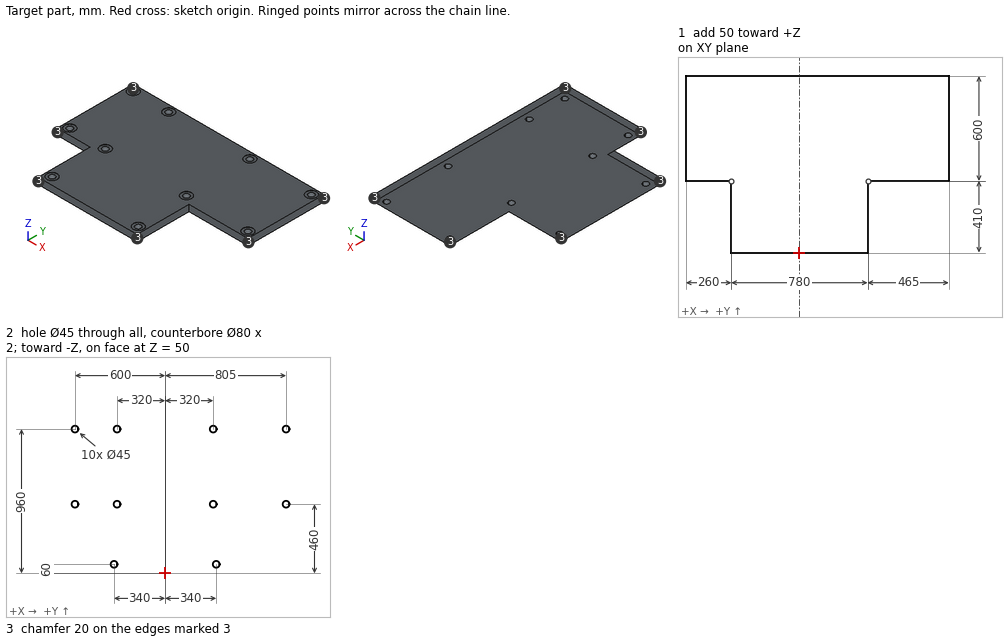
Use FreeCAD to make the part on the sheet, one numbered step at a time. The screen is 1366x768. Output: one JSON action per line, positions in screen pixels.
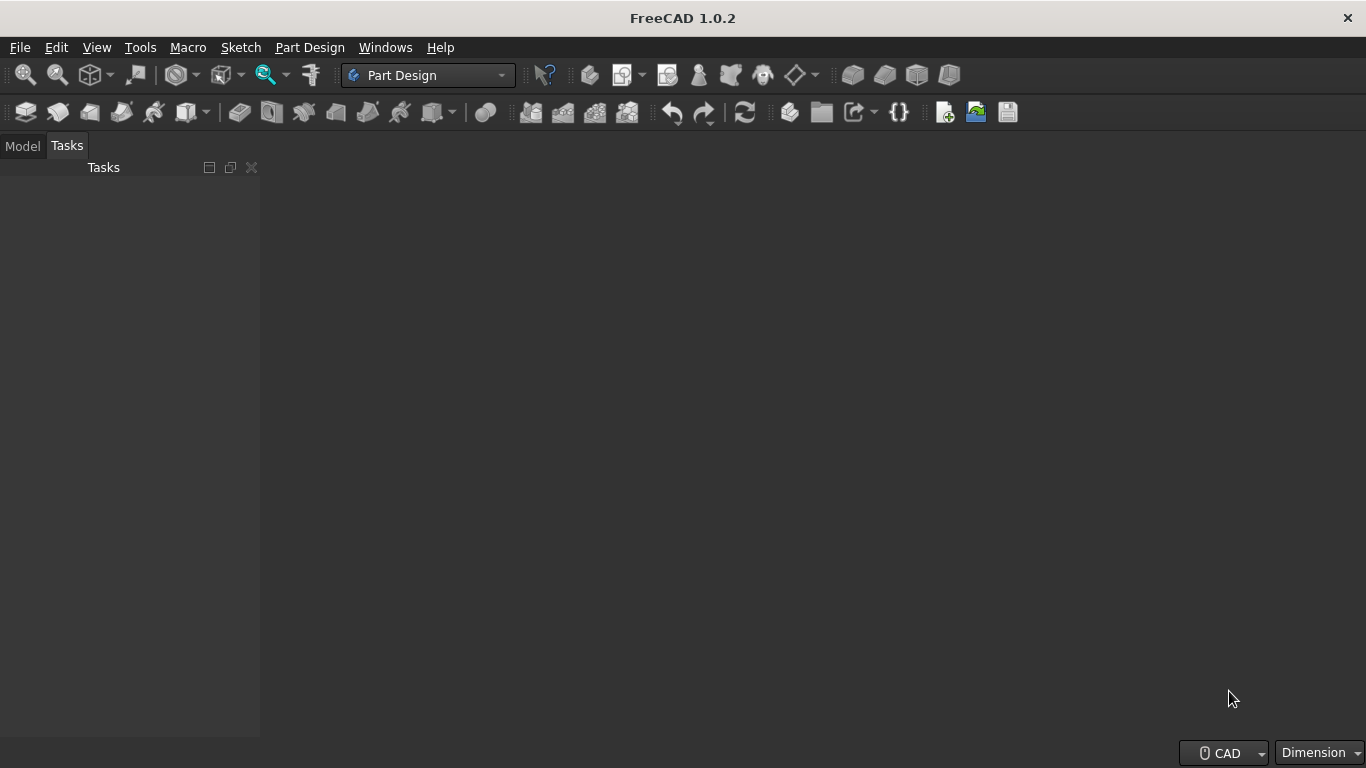
{"action": "left_click", "coordinate": [944, 112]}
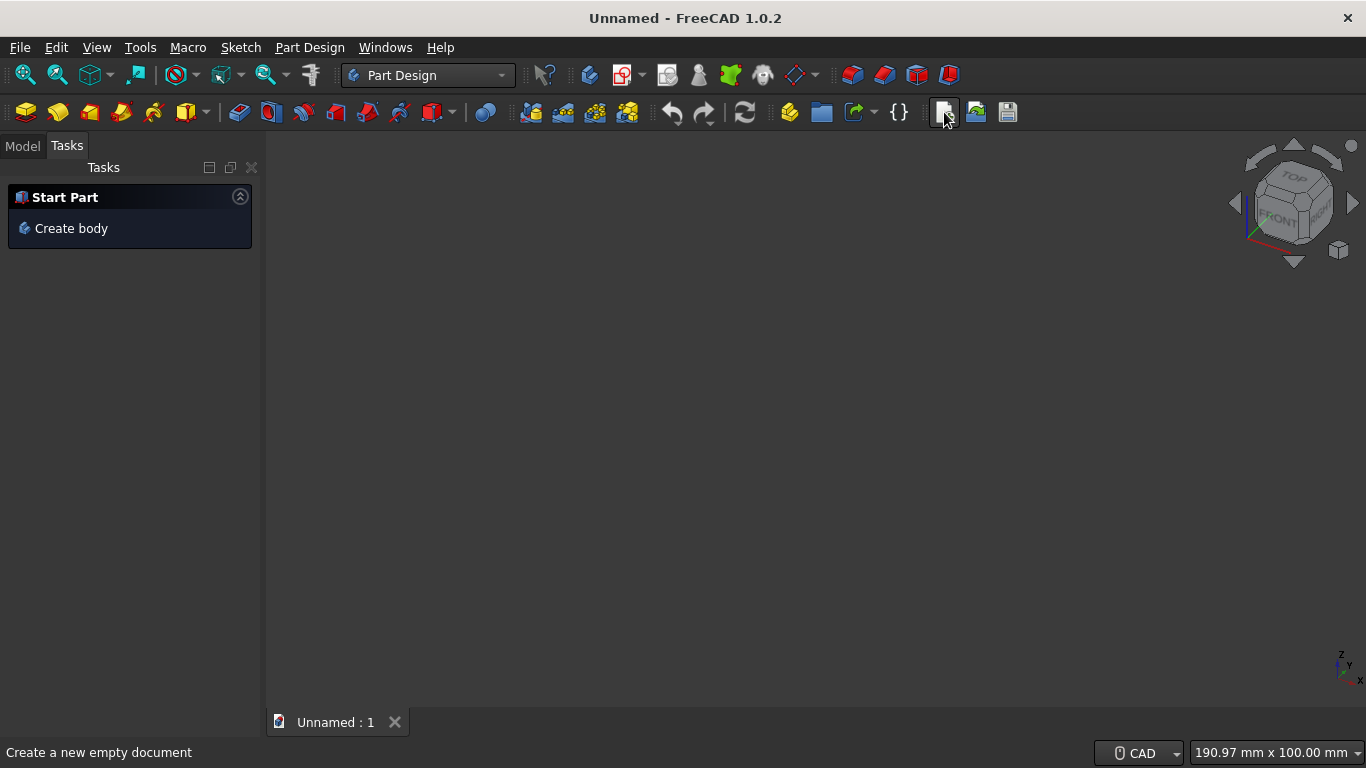
{"action": "left_click", "coordinate": [622, 76]}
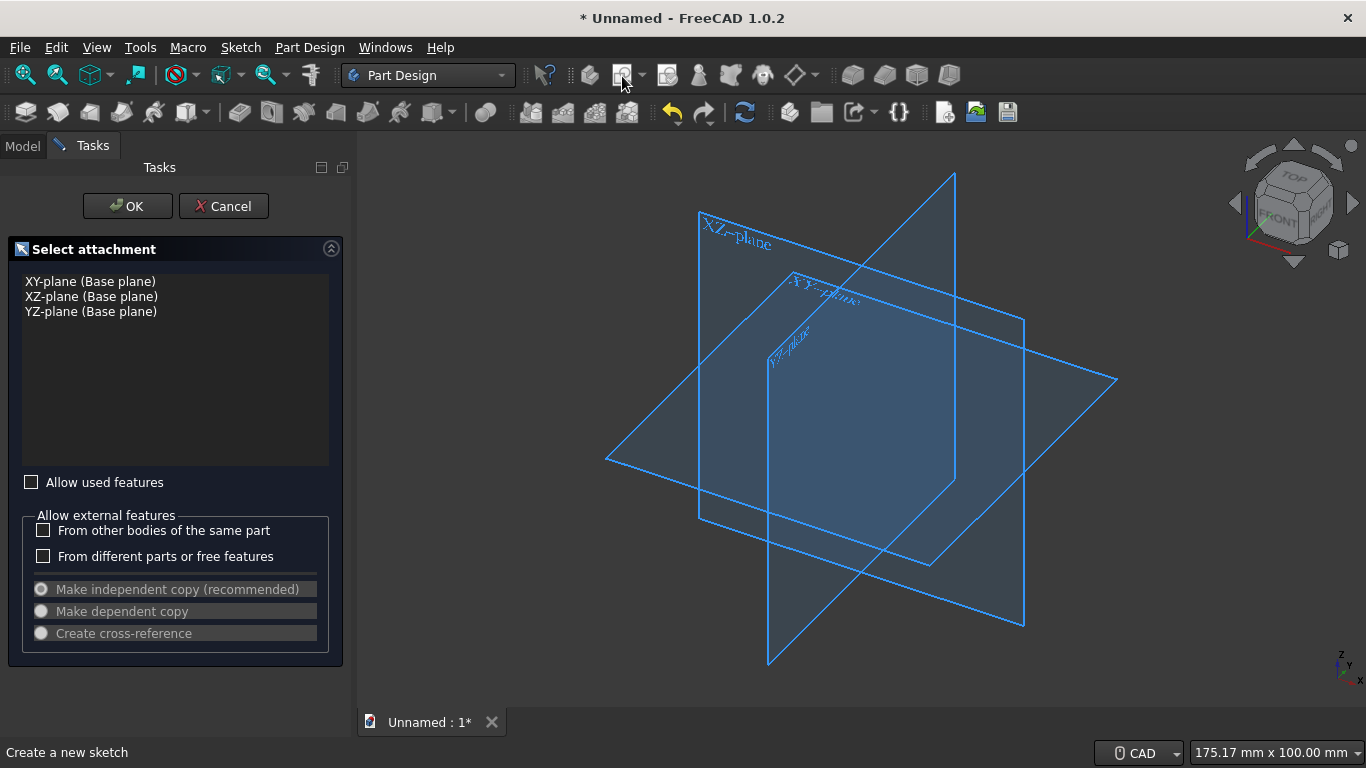
{"action": "left_click", "coordinate": [82, 282]}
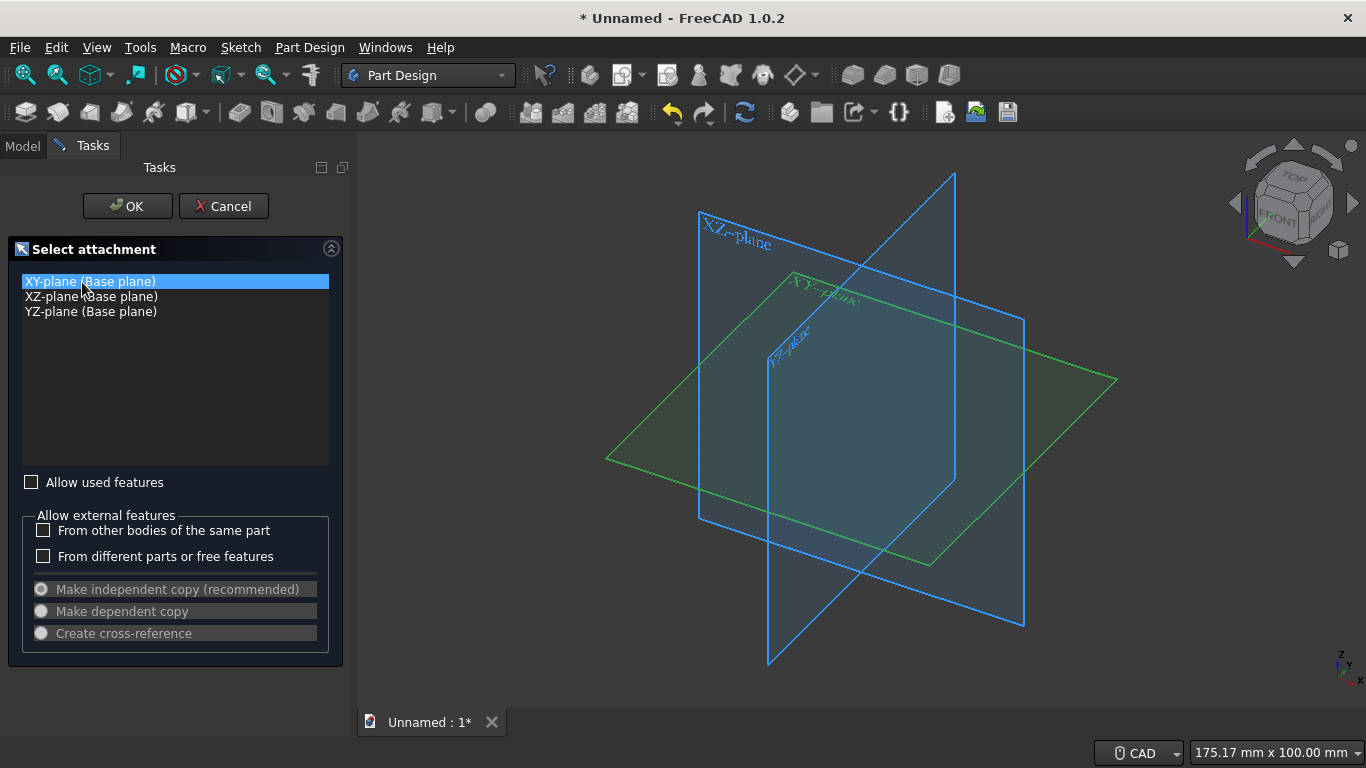
{"action": "left_click", "coordinate": [128, 206]}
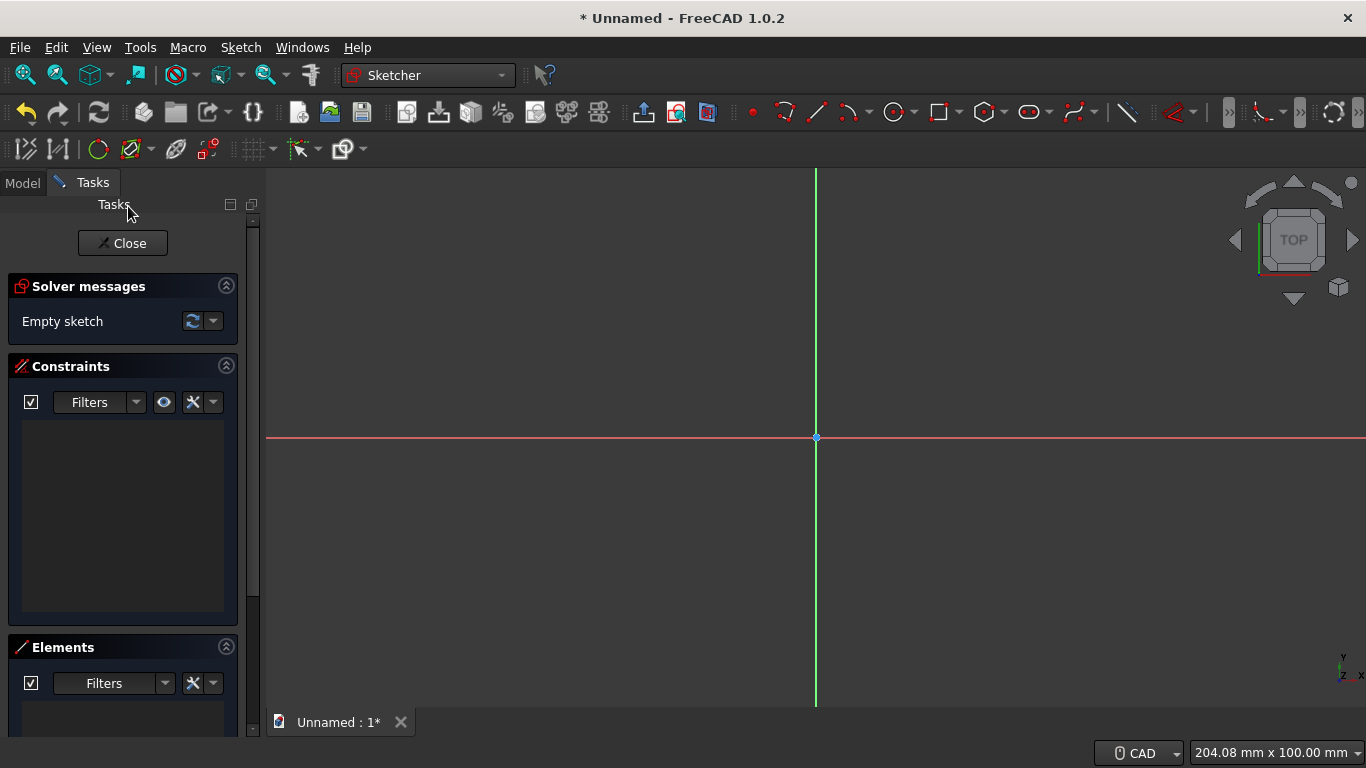
{"action": "scroll", "coordinate": [707, 614], "scroll_direction": "down", "scroll_amount": 14}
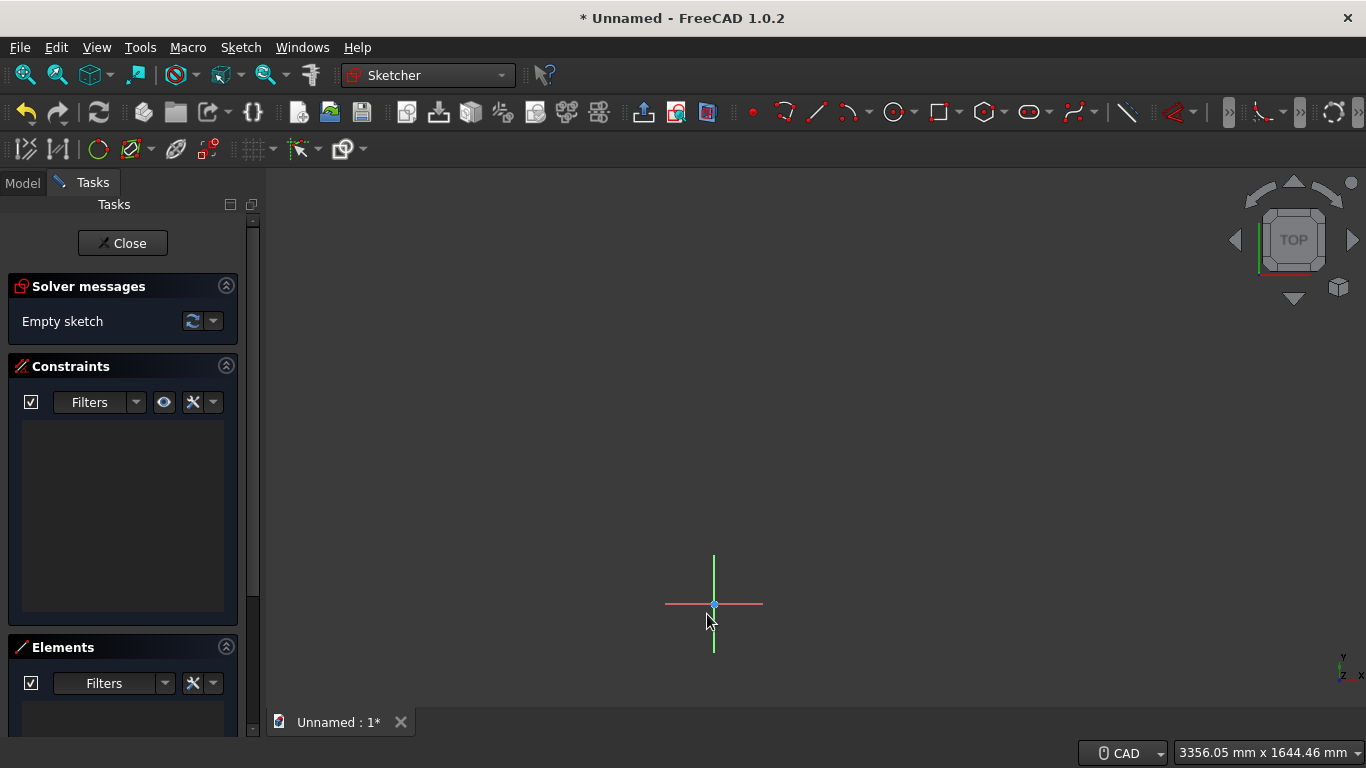
{"action": "left_click", "coordinate": [786, 112]}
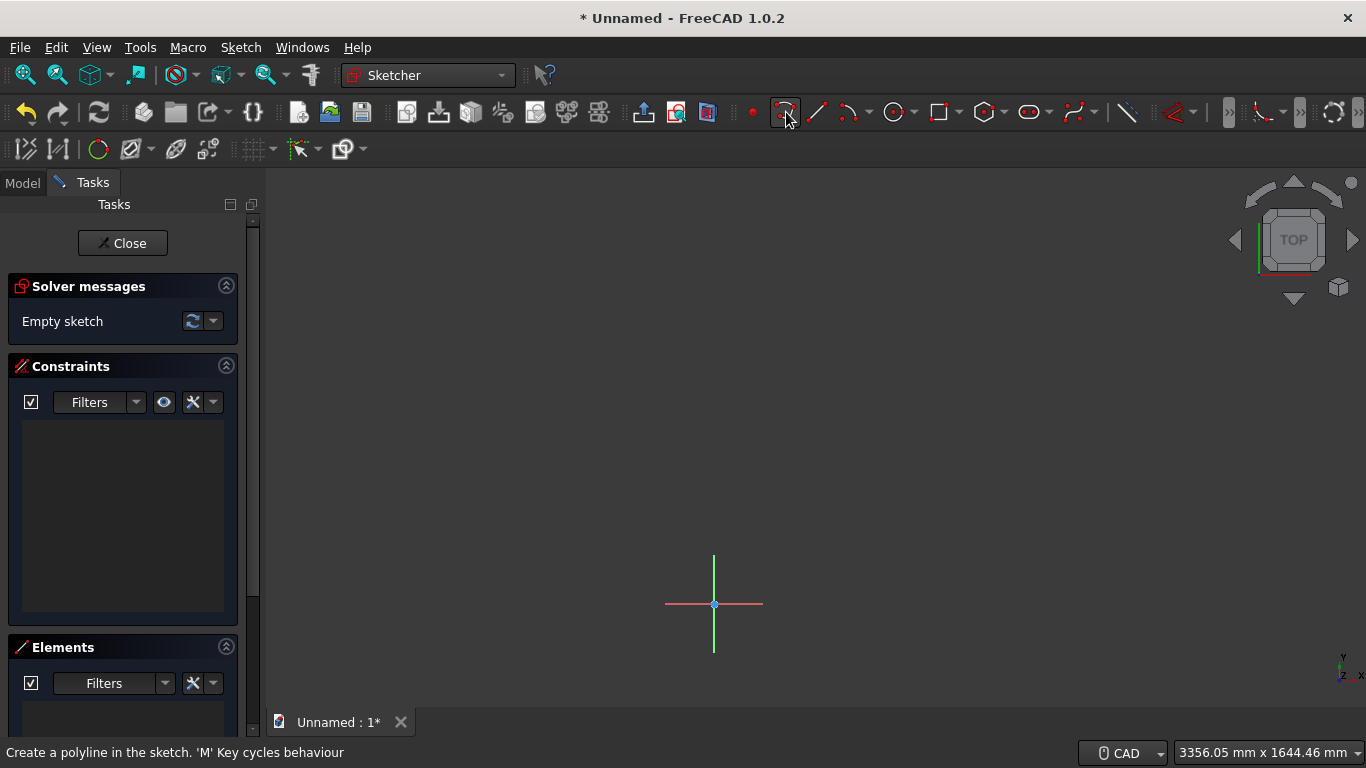
{"action": "left_click", "coordinate": [586, 604]}
{"action": "left_click", "coordinate": [842, 595]}
{"action": "left_click", "coordinate": [842, 470]}
{"action": "left_click", "coordinate": [994, 470]}
{"action": "left_click", "coordinate": [994, 273]}
{"action": "left_click", "coordinate": [501, 273]}
{"action": "left_click", "coordinate": [501, 470]}
{"action": "left_click", "coordinate": [586, 470]}
{"action": "left_click", "coordinate": [586, 605]}
{"action": "key", "text": "Escape"}
{"action": "key", "text": "Escape"}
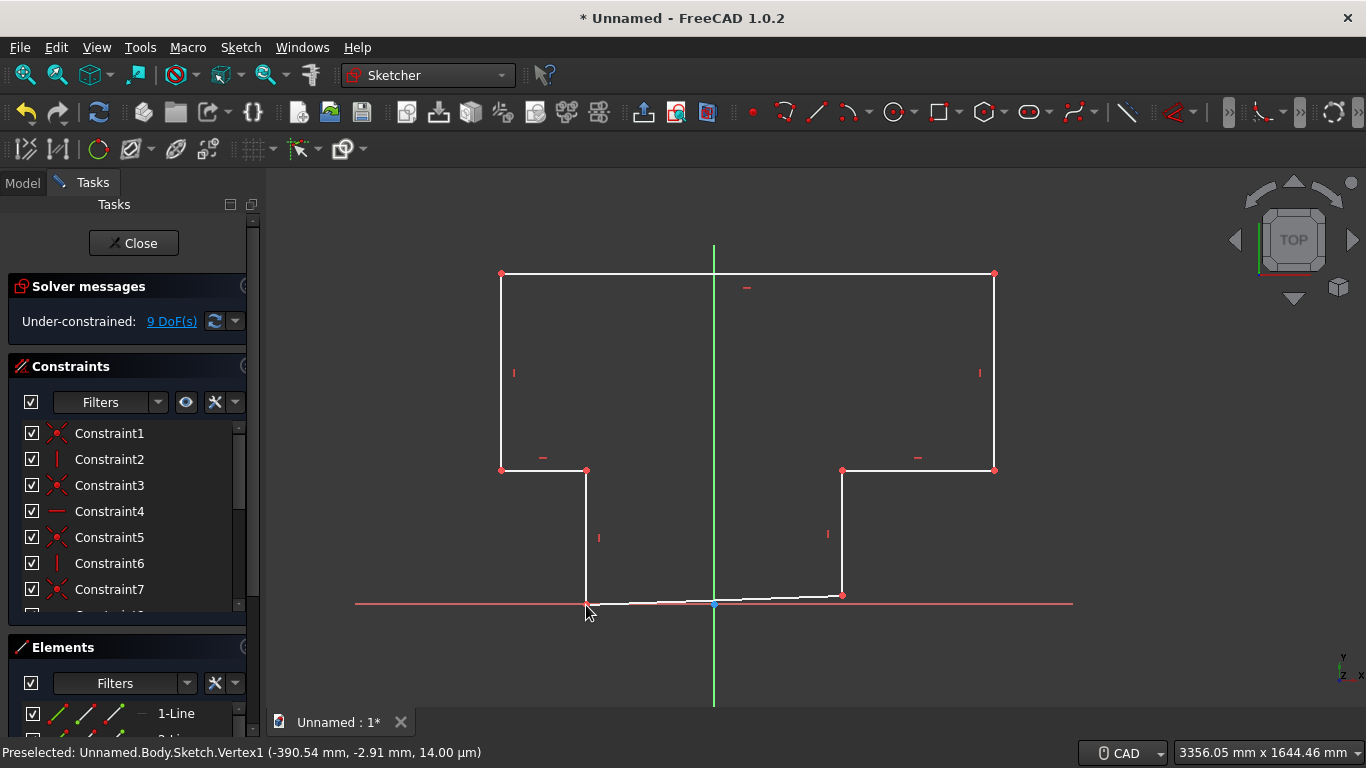
{"action": "left_click", "coordinate": [663, 602]}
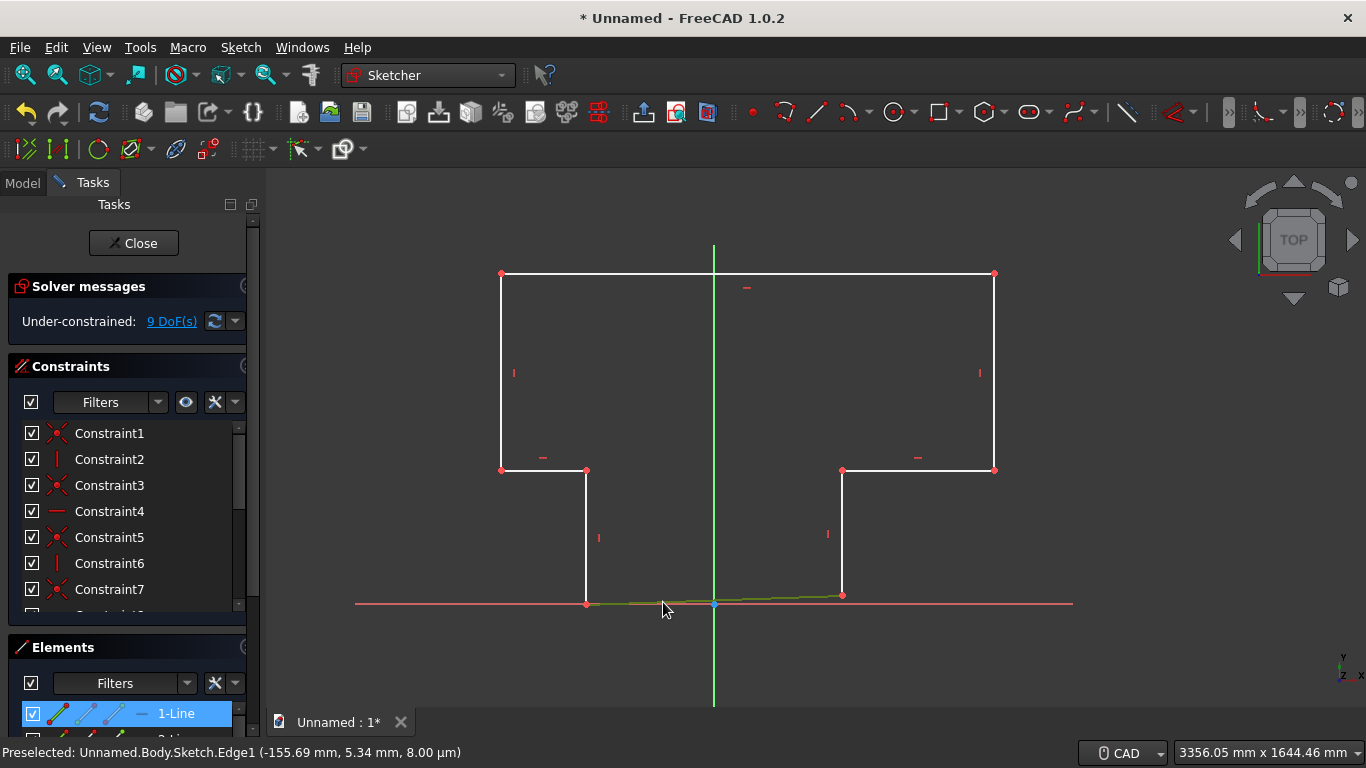
{"action": "key", "text": "h"}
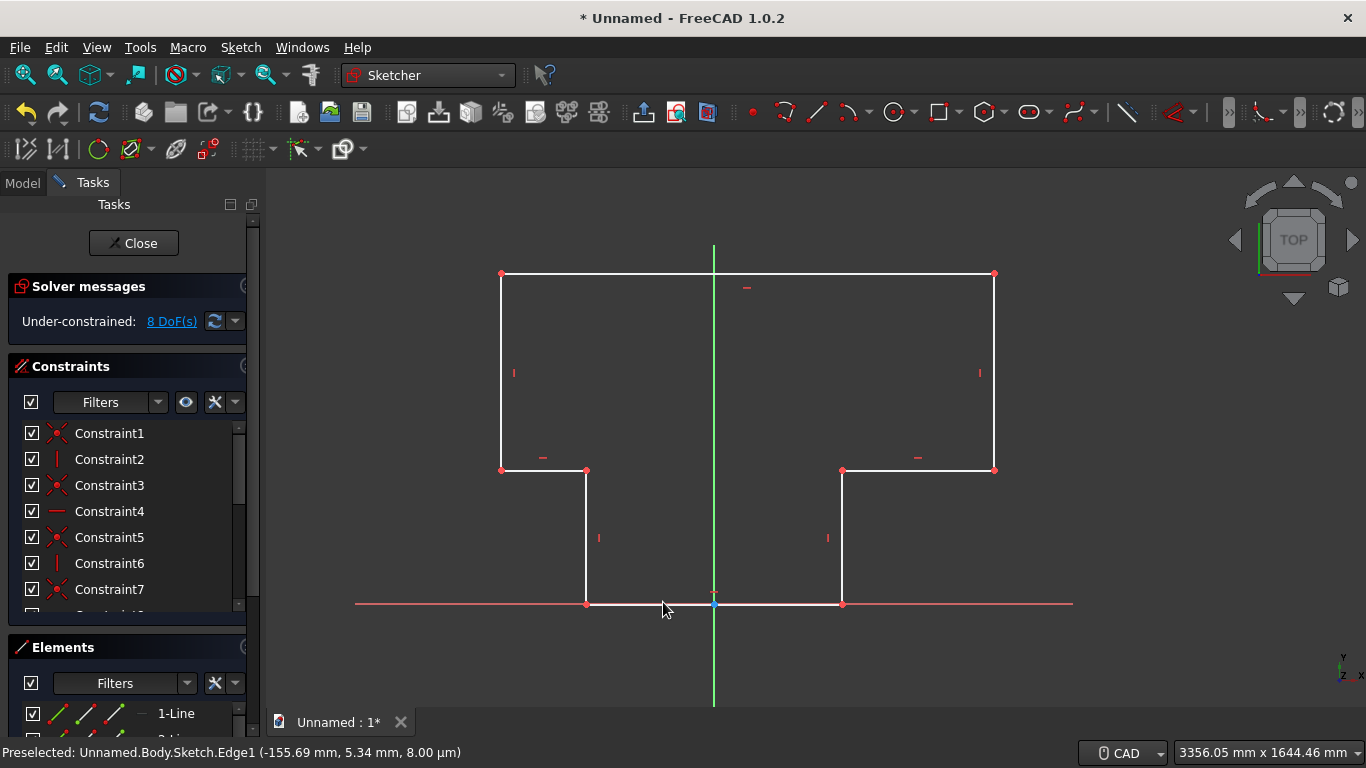
{"action": "left_click", "coordinate": [842, 471]}